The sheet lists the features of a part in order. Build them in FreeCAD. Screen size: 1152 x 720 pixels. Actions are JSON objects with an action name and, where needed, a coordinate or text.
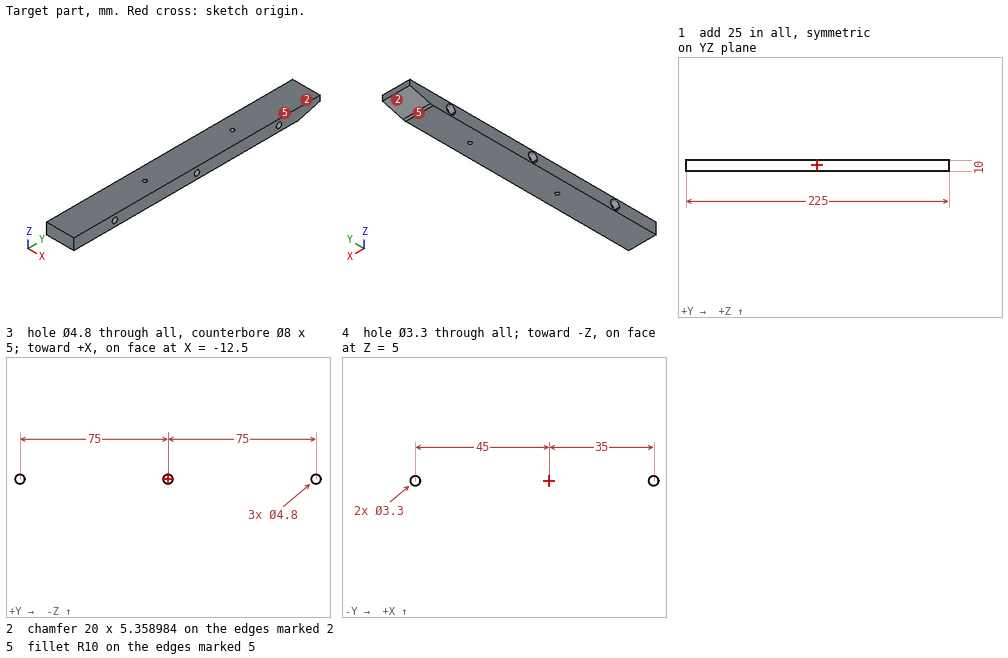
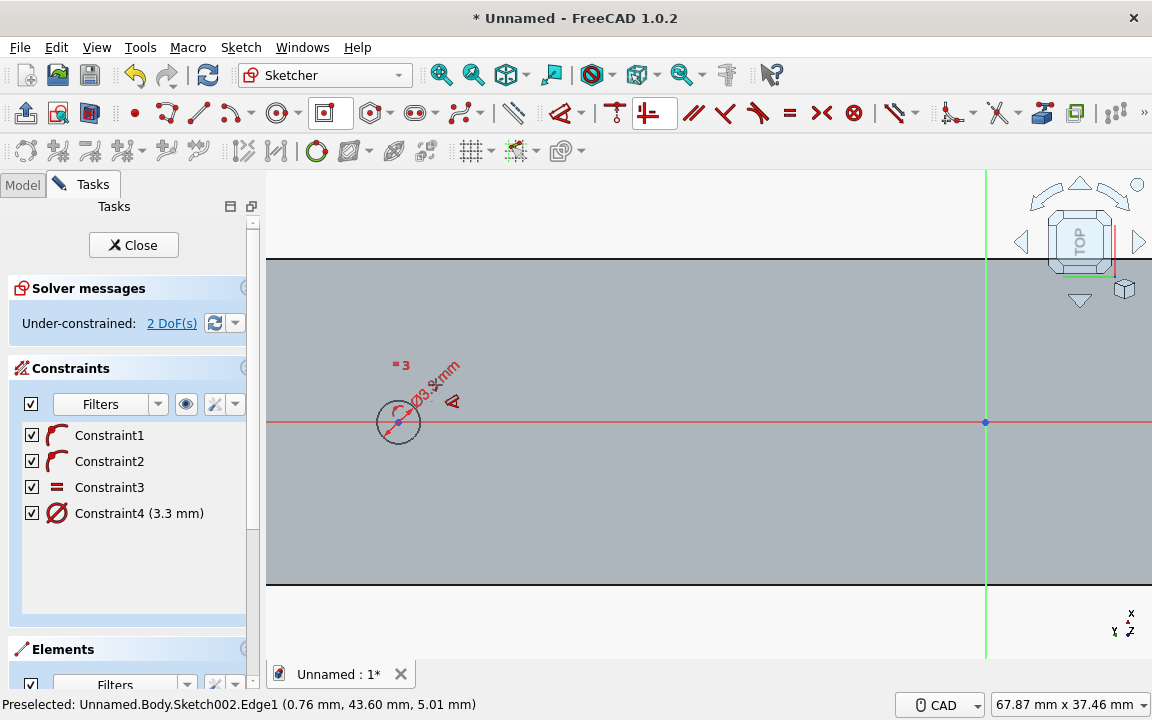
{"action": "left_click", "coordinate": [399, 422]}
{"action": "left_click", "coordinate": [692, 456]}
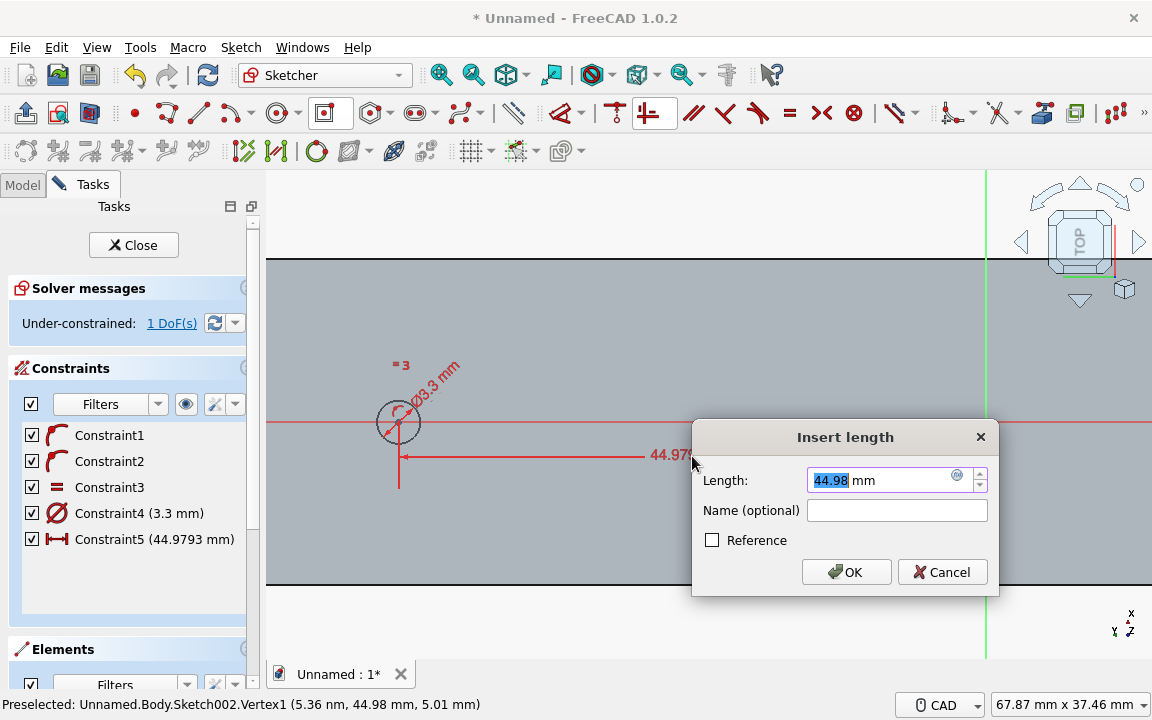
{"action": "type", "text": "45"}
{"action": "key", "text": "Return"}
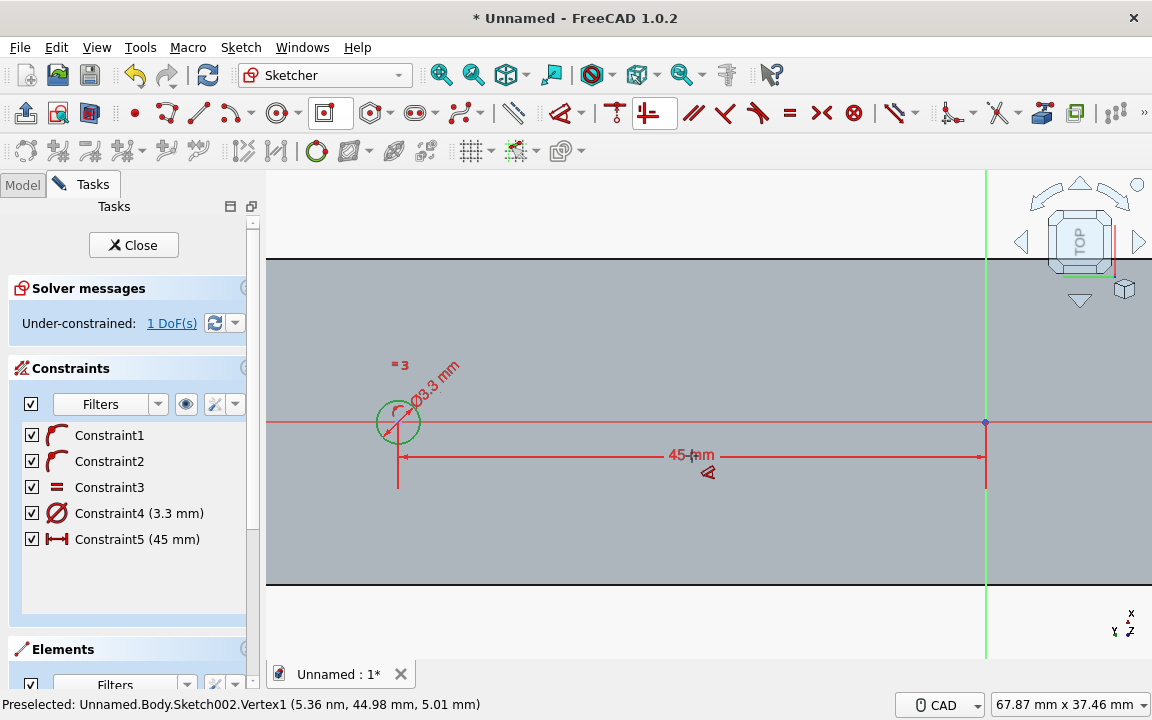
{"action": "scroll", "coordinate": [412, 408], "scroll_direction": "down", "scroll_amount": 4}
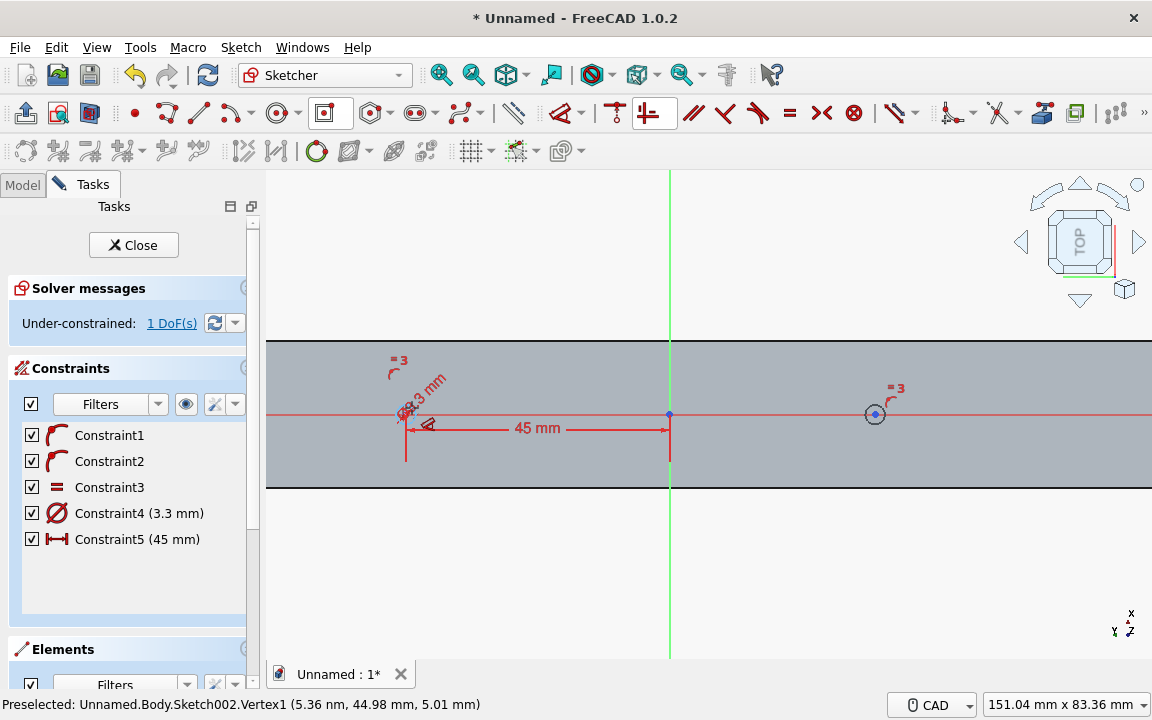
{"action": "left_click", "coordinate": [875, 415]}
{"action": "left_click", "coordinate": [773, 381]}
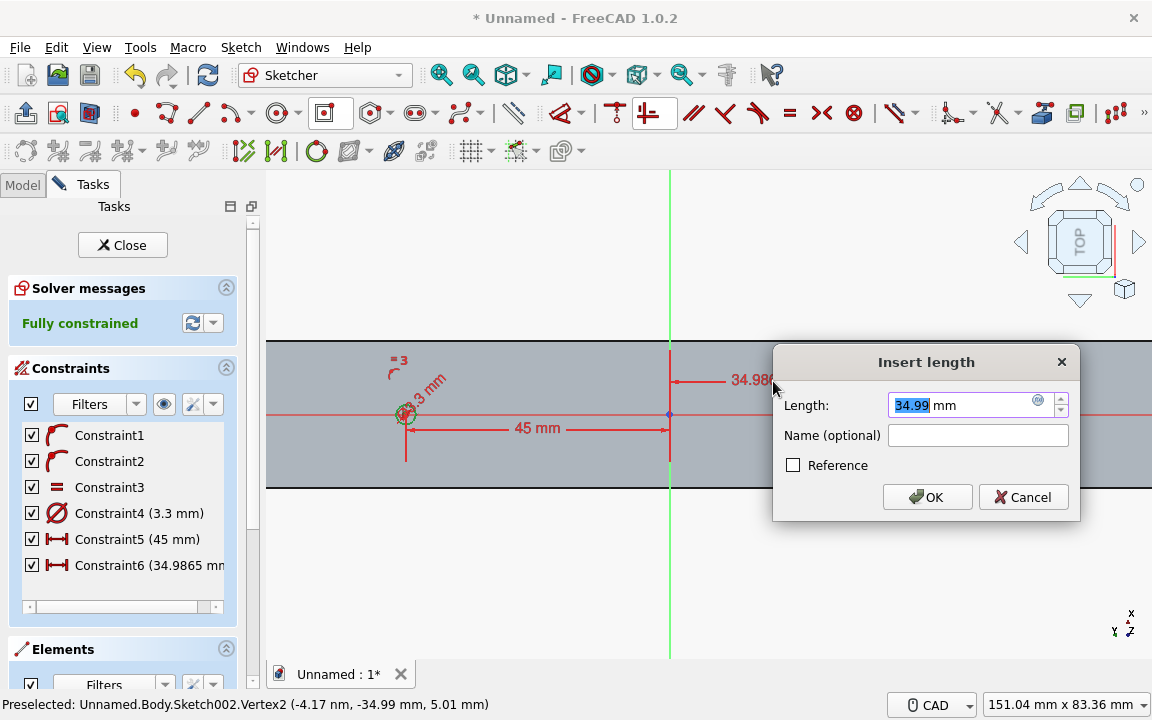
{"action": "type", "text": "35"}
{"action": "key", "text": "Return"}
{"action": "key", "text": "Escape"}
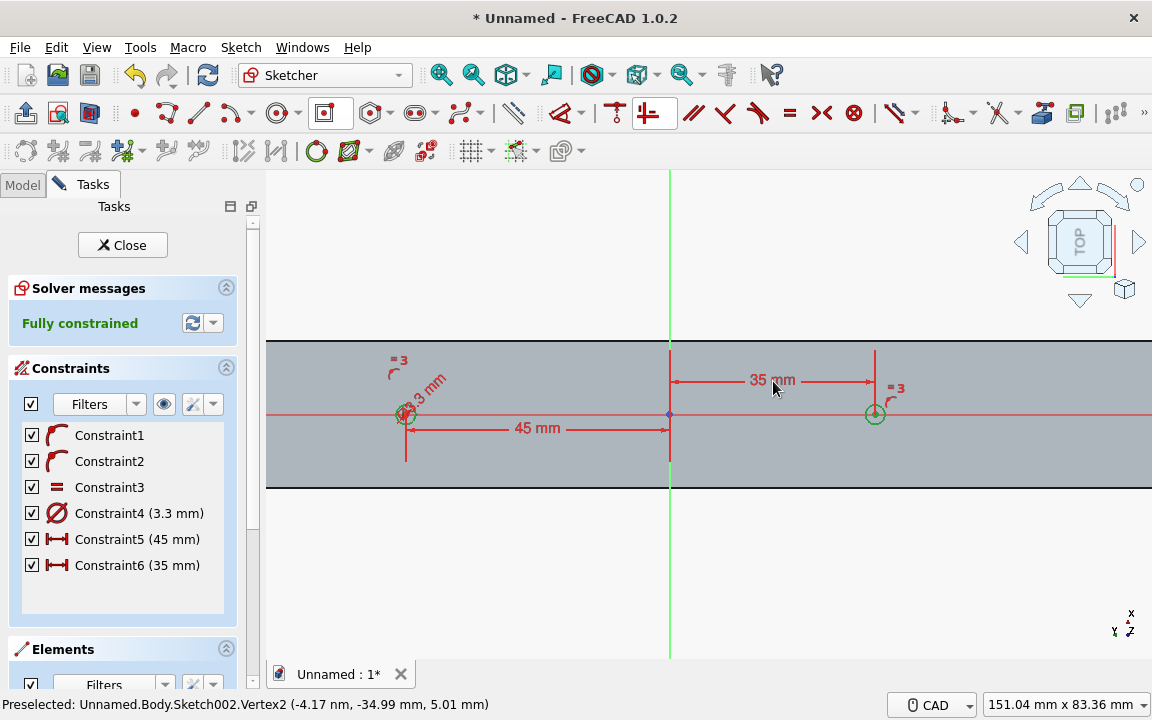
{"action": "left_click", "coordinate": [123, 245]}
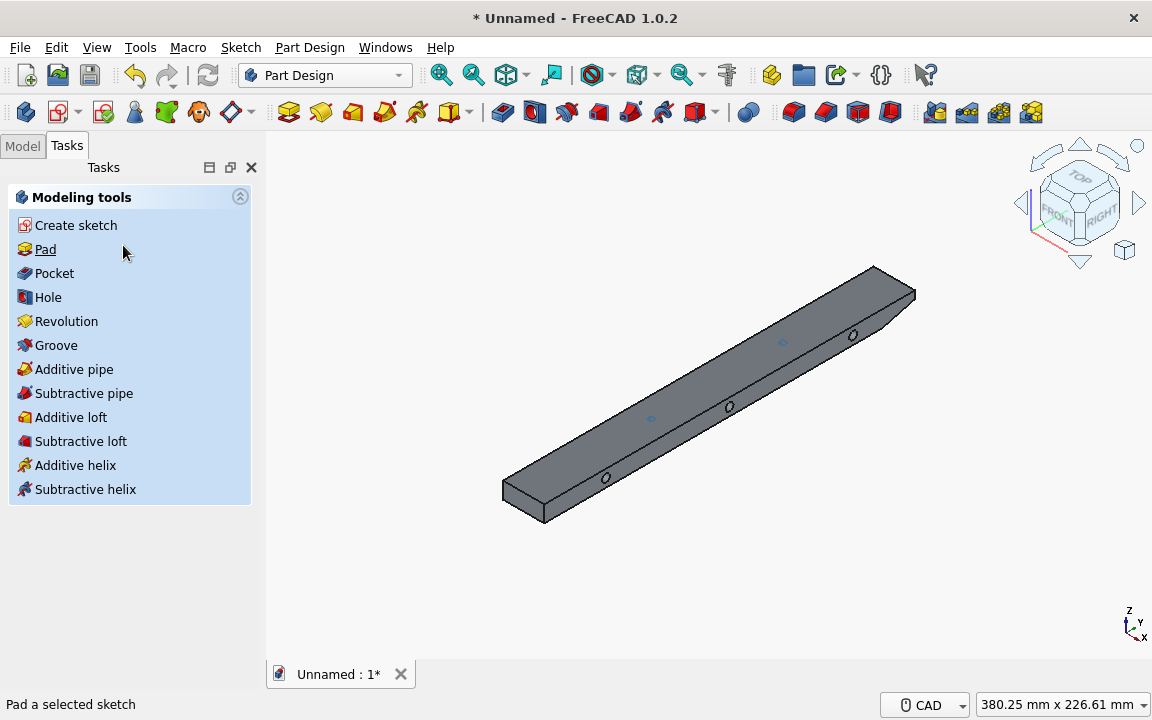
{"action": "left_click", "coordinate": [536, 112]}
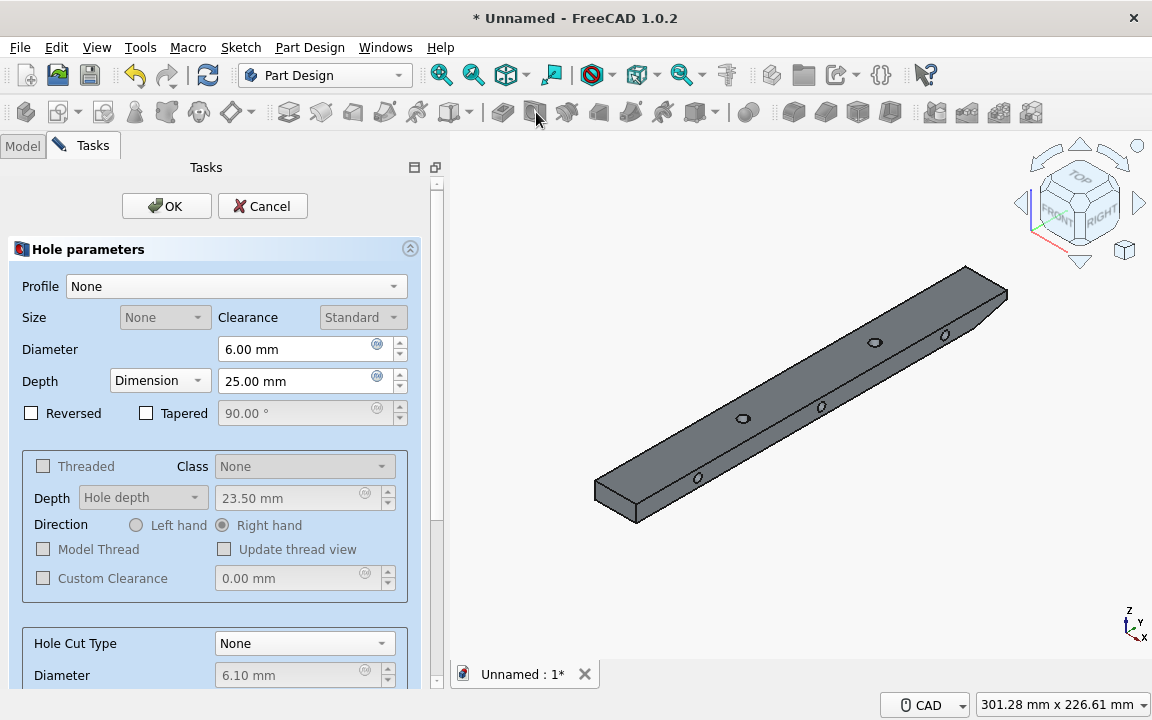
{"action": "triple_click", "coordinate": [305, 349]}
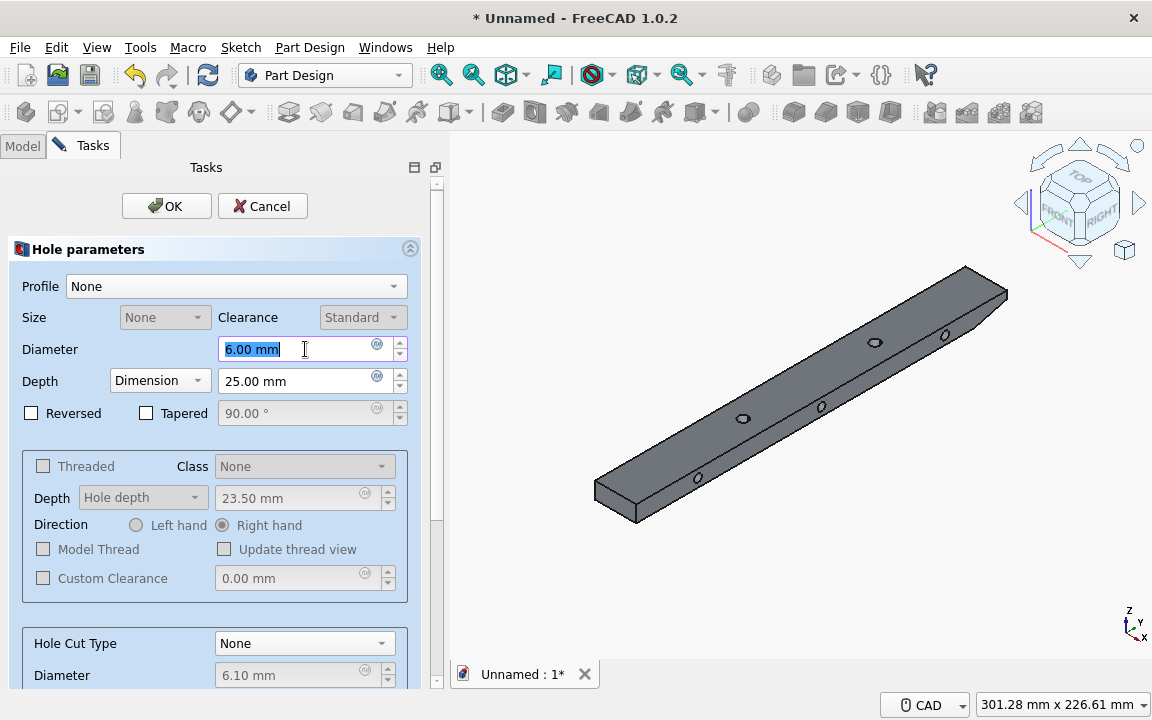
{"action": "type", "text": "3.3"}
{"action": "key", "text": "Tab"}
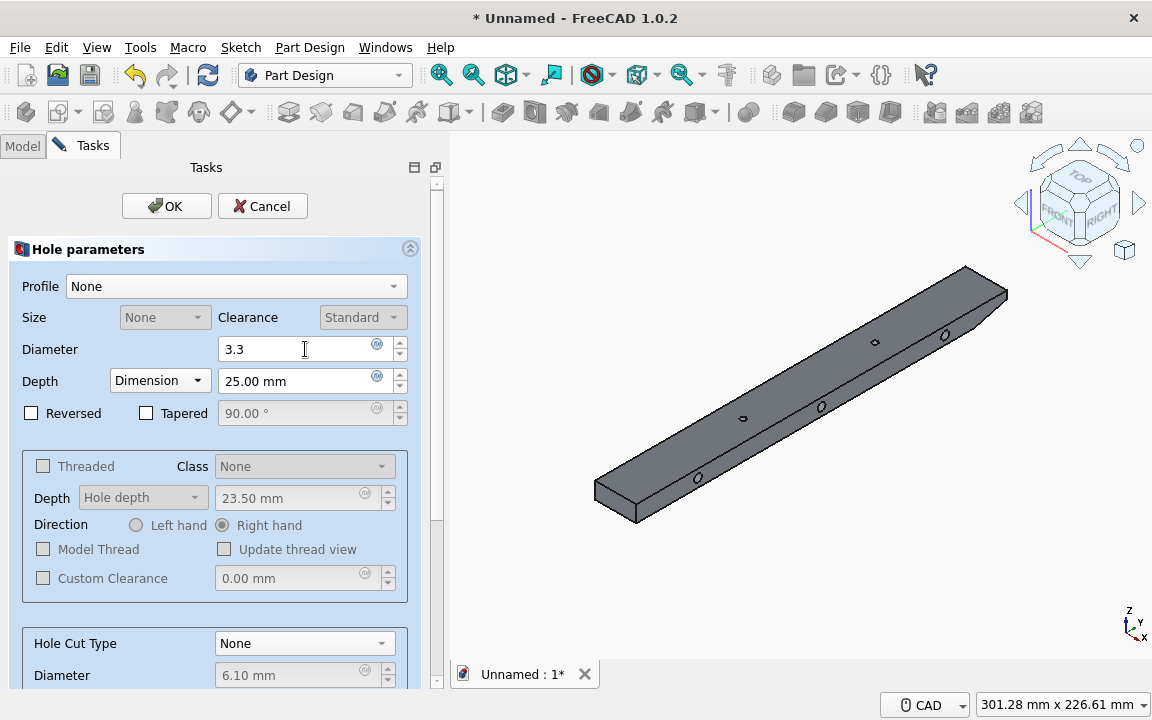
{"action": "left_click", "coordinate": [161, 380]}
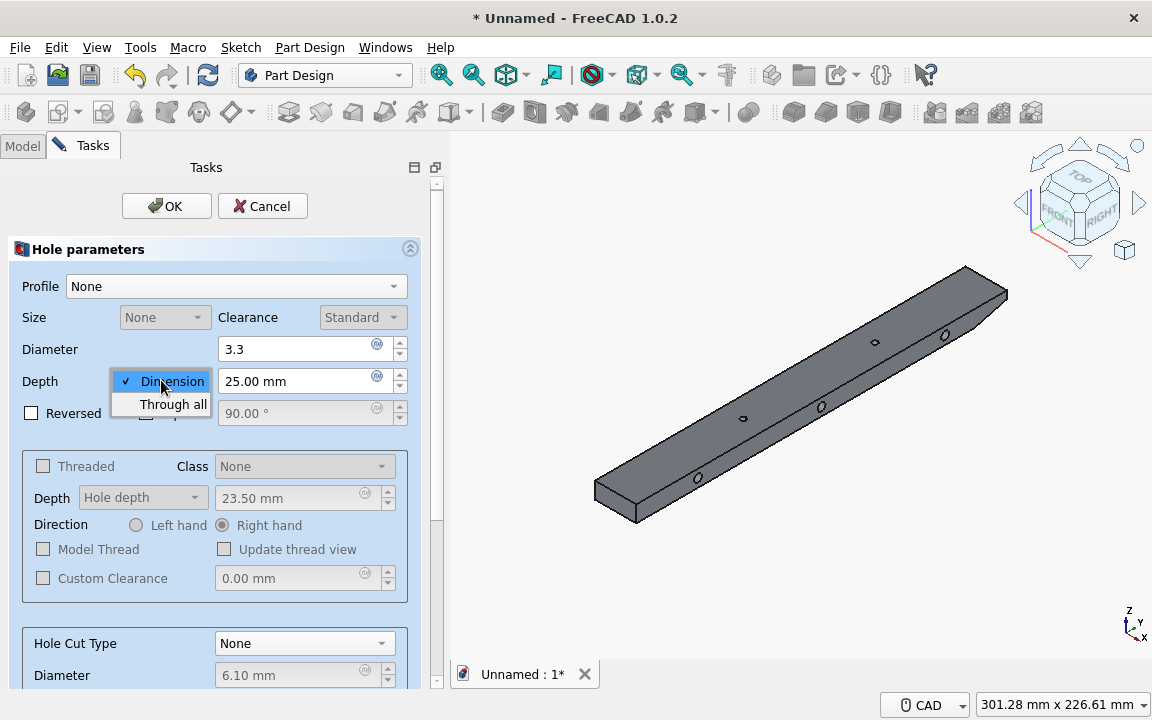
{"action": "left_click", "coordinate": [160, 404]}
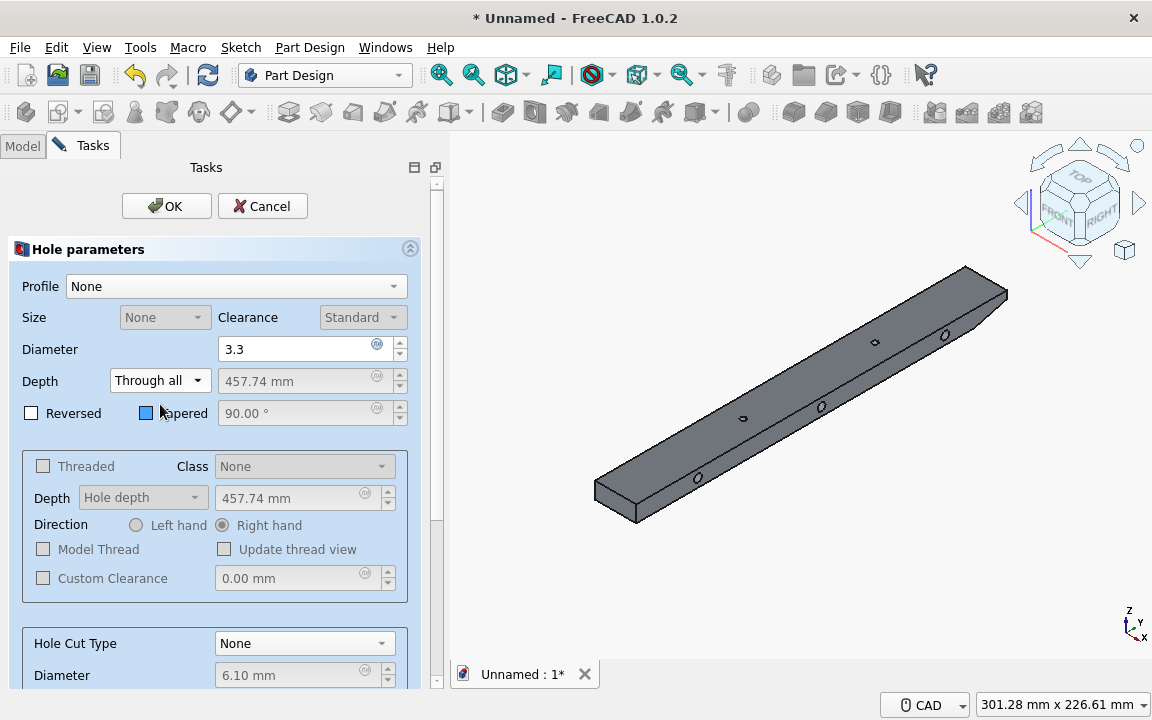
{"action": "left_click", "coordinate": [167, 206]}